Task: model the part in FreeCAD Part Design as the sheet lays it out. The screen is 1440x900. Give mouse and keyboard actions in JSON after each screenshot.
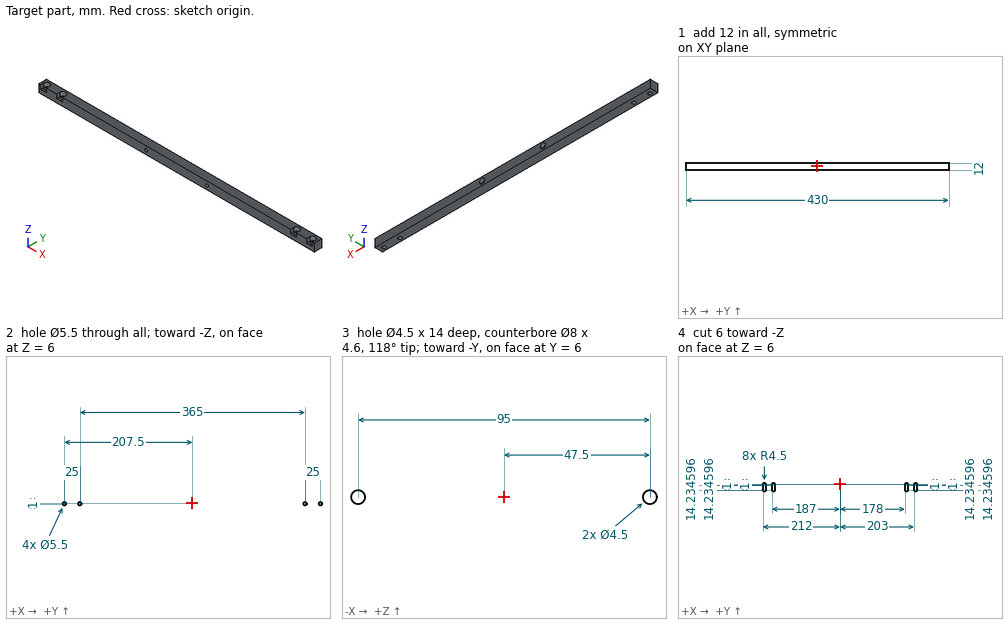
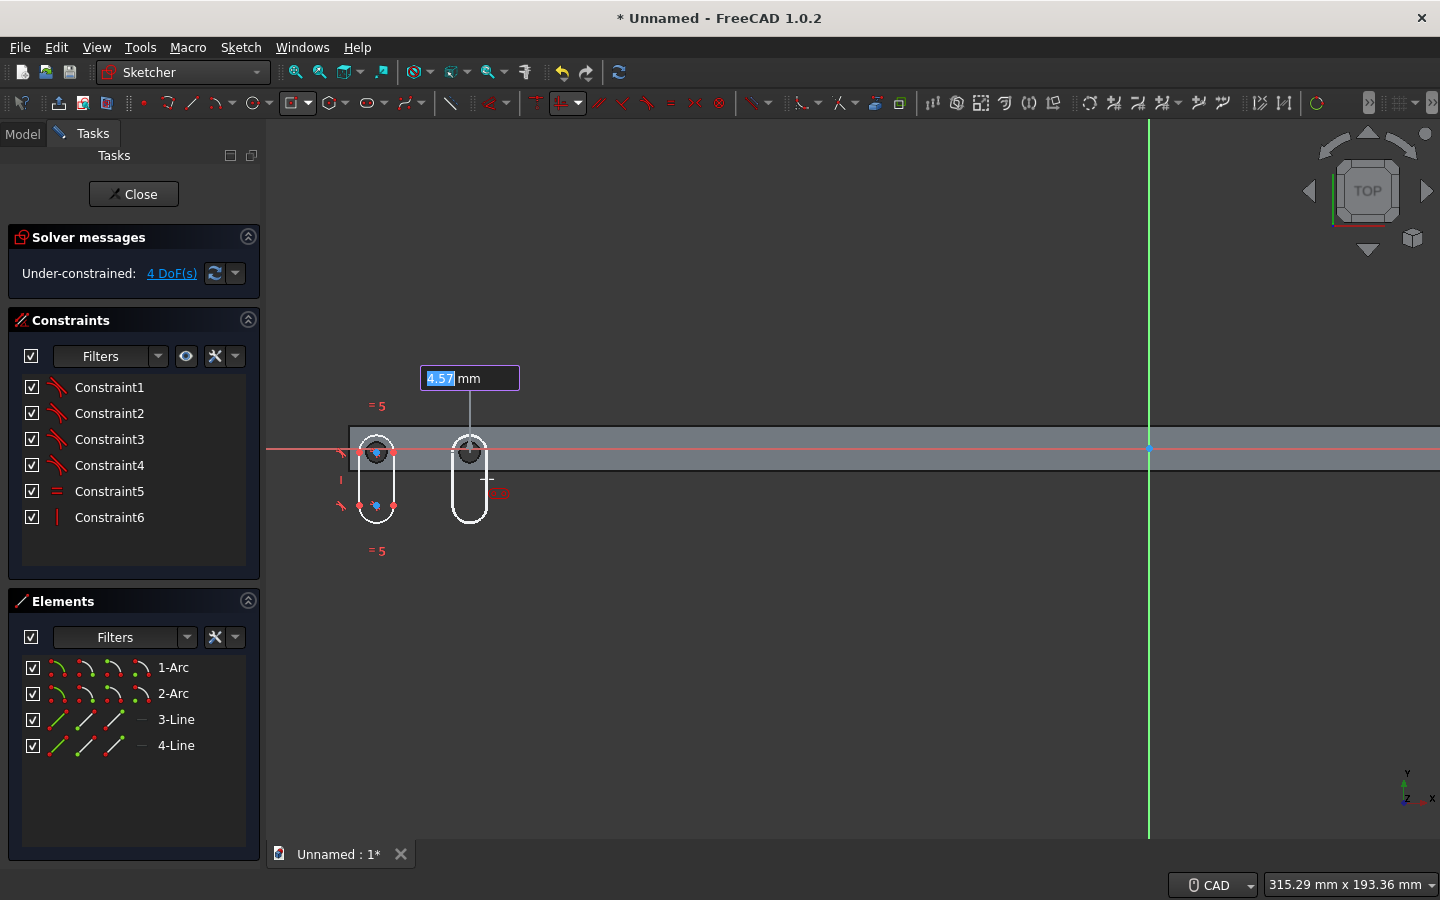
{"action": "left_click", "coordinate": [486, 479]}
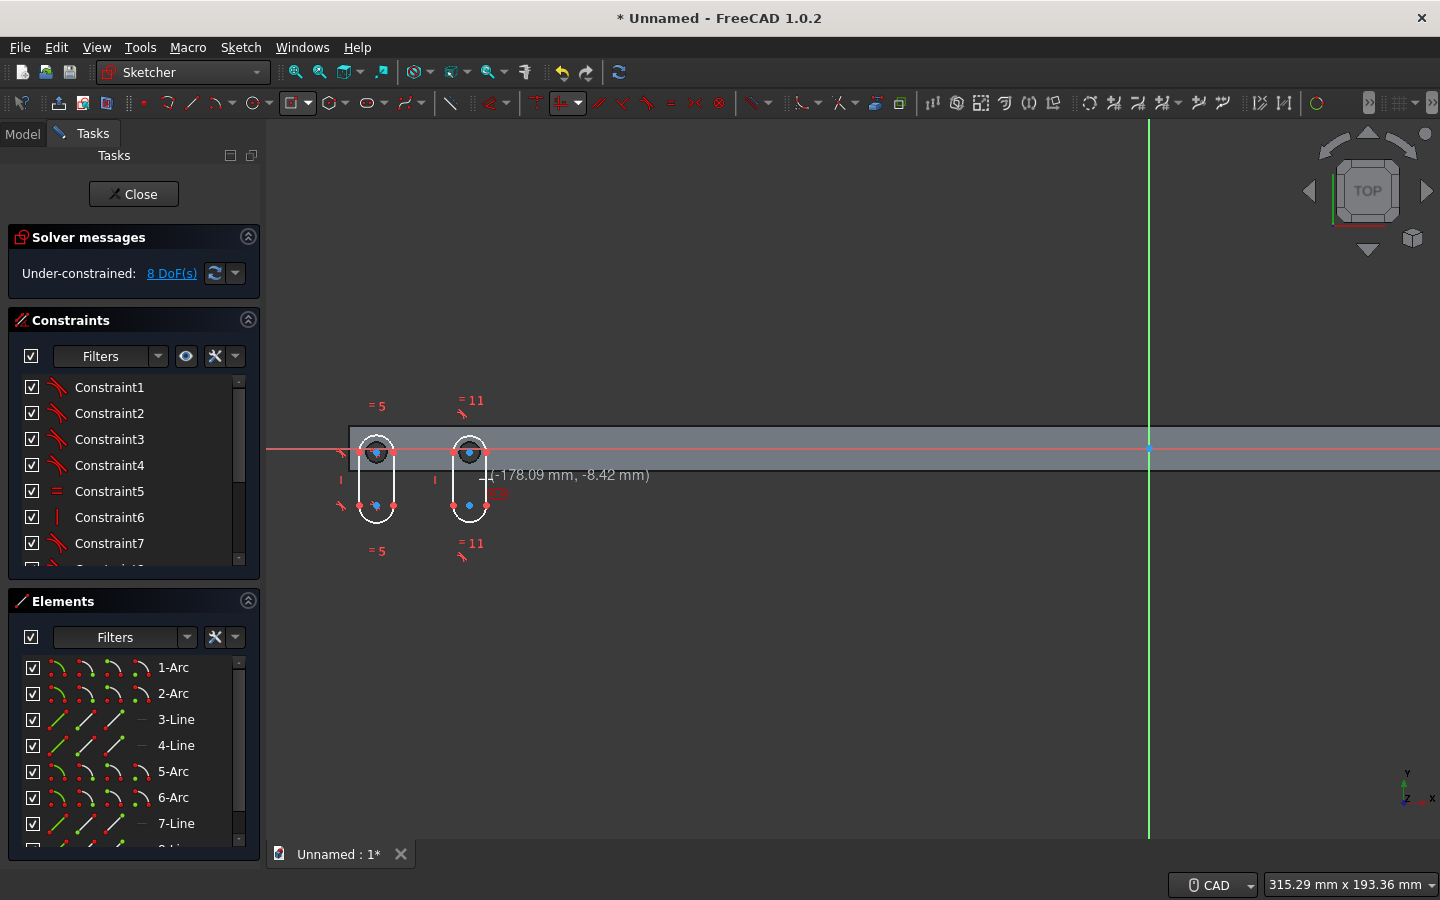
{"action": "scroll", "coordinate": [487, 479], "scroll_direction": "down", "scroll_amount": 4}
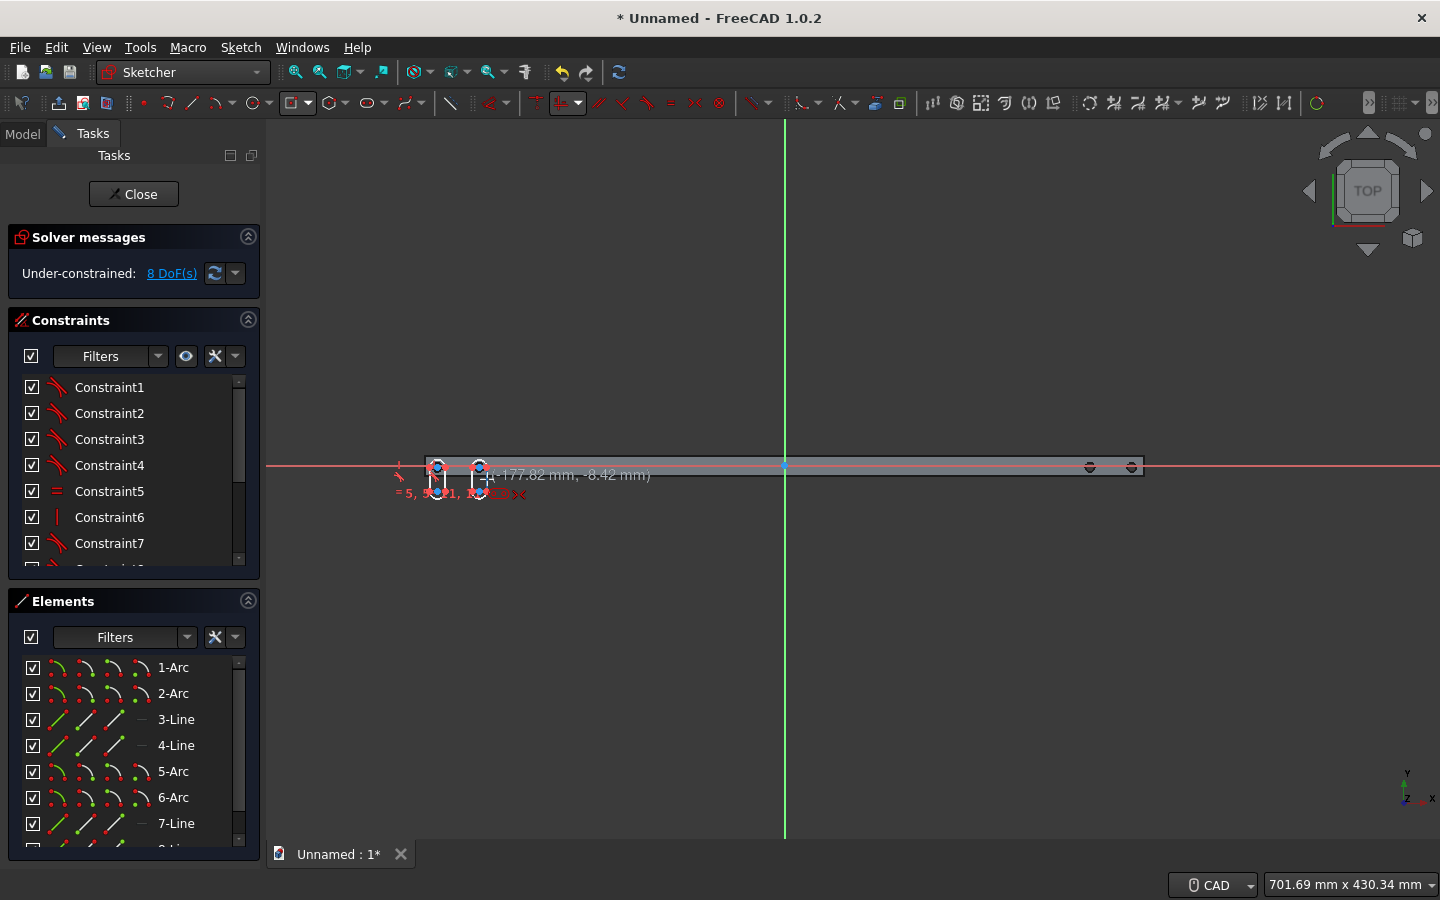
{"action": "scroll", "coordinate": [1090, 491], "scroll_direction": "up", "scroll_amount": 6}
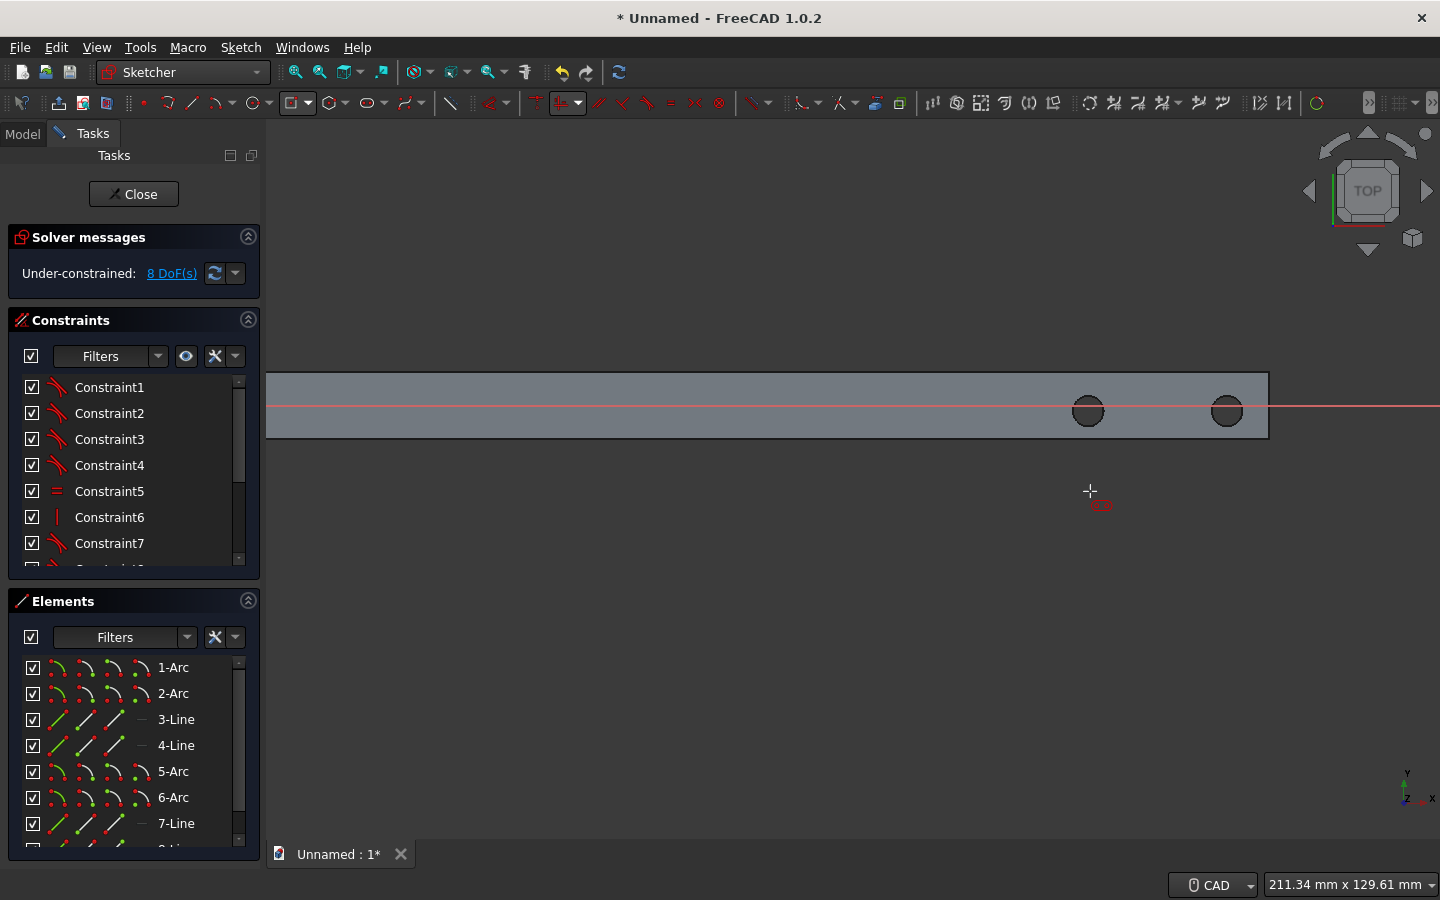
{"action": "left_click", "coordinate": [1088, 490]}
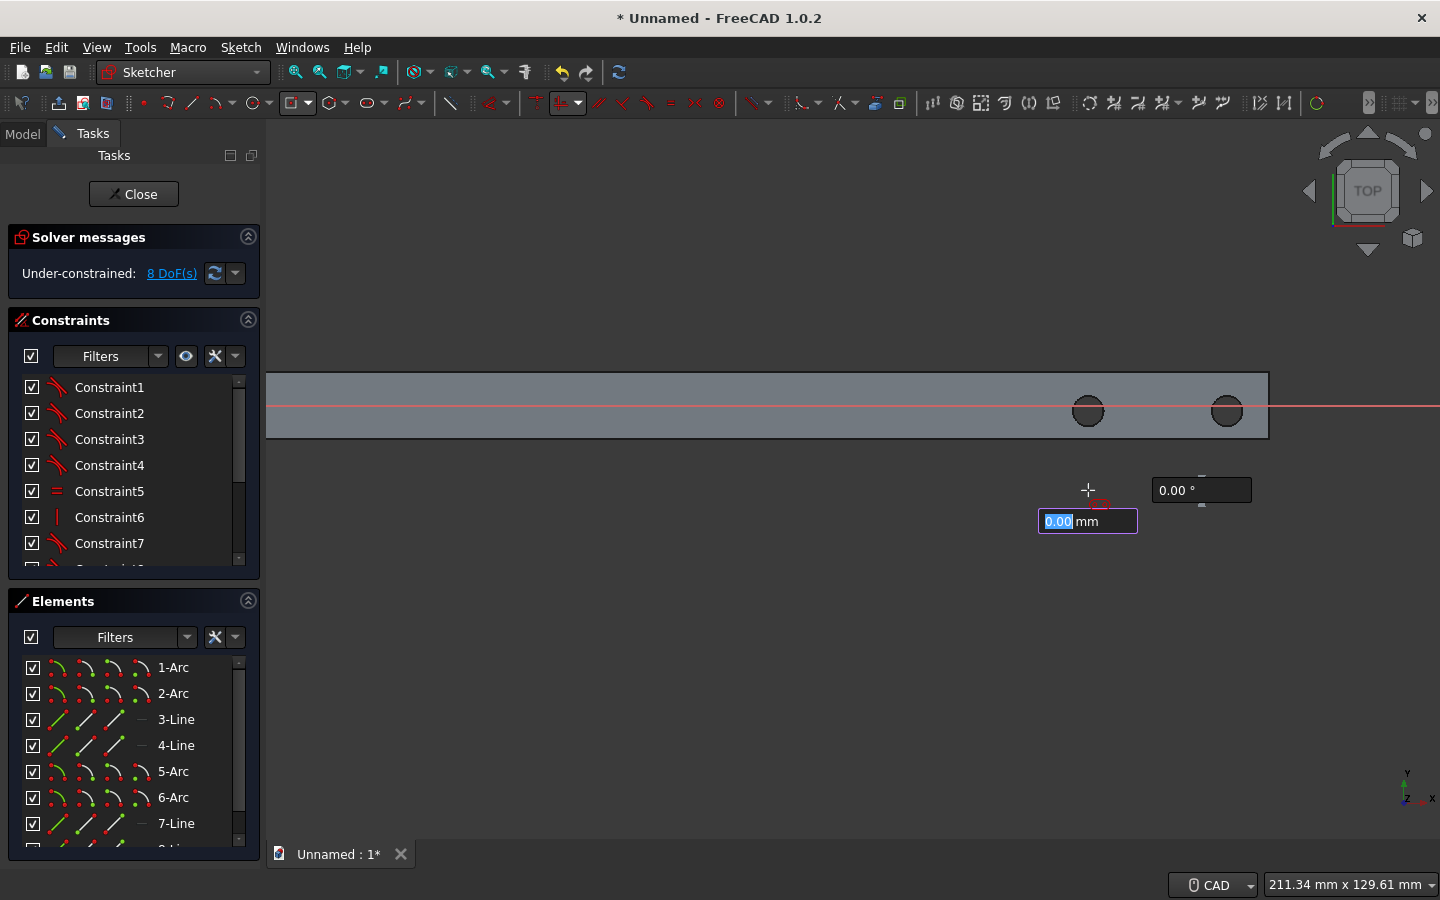
{"action": "scroll", "coordinate": [1088, 411], "scroll_direction": "up", "scroll_amount": 6}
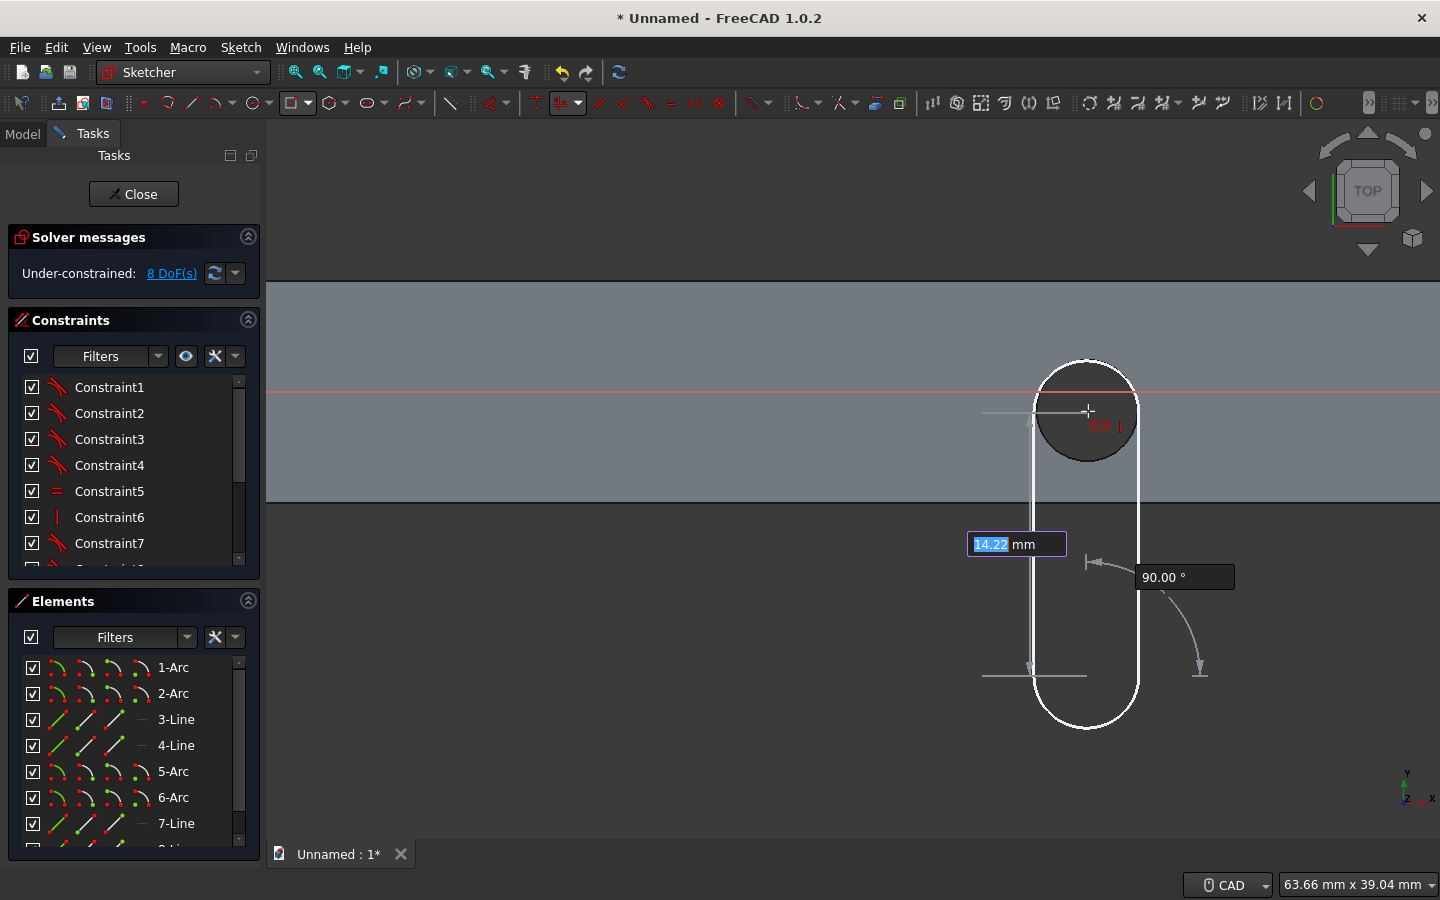
{"action": "left_click", "coordinate": [1086, 410]}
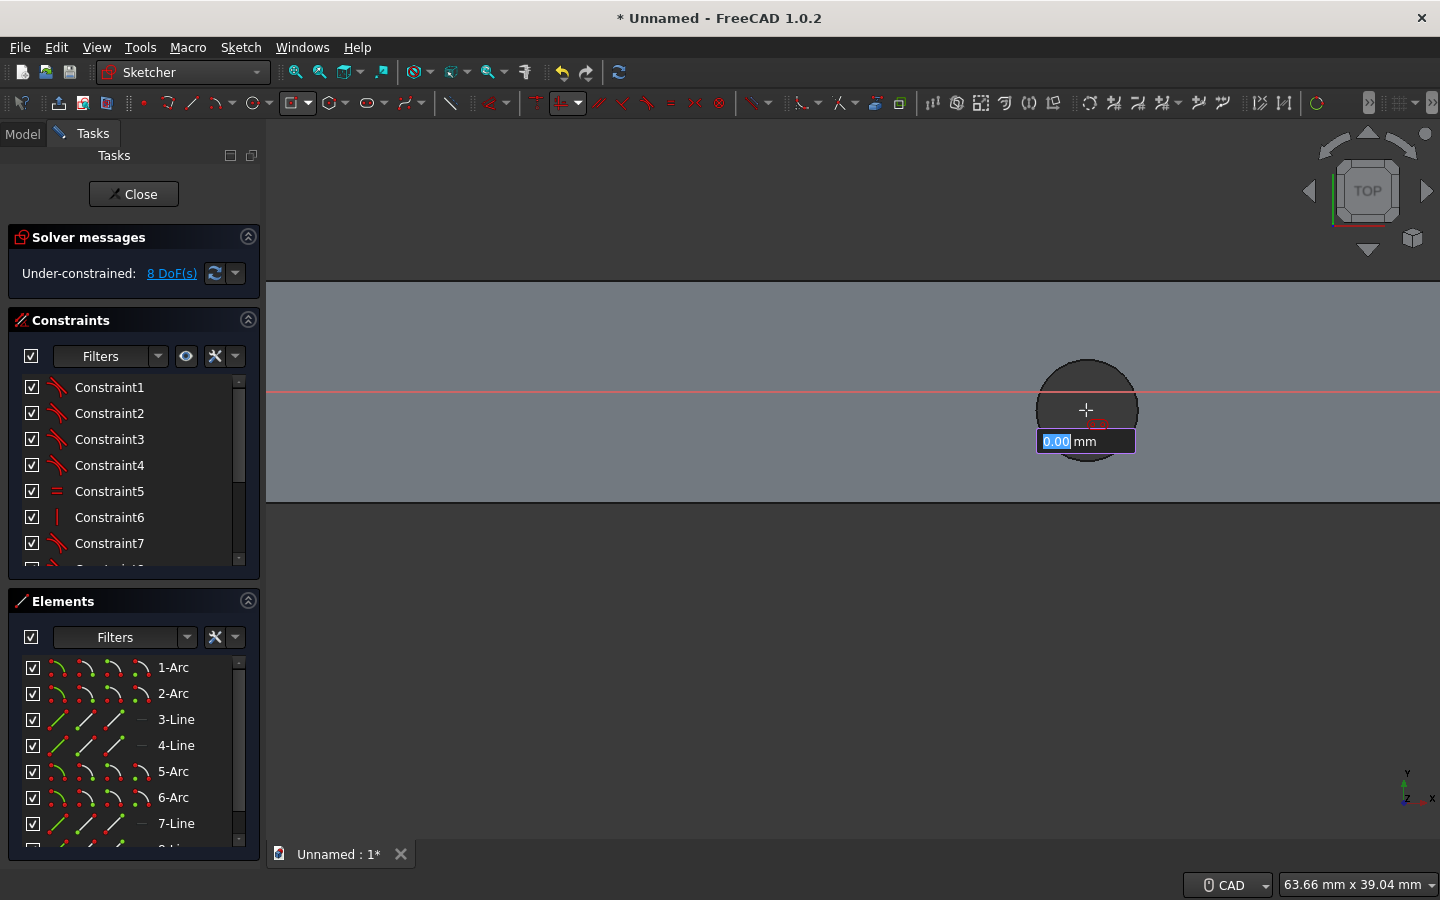
{"action": "scroll", "coordinate": [1090, 473], "scroll_direction": "down", "scroll_amount": 12}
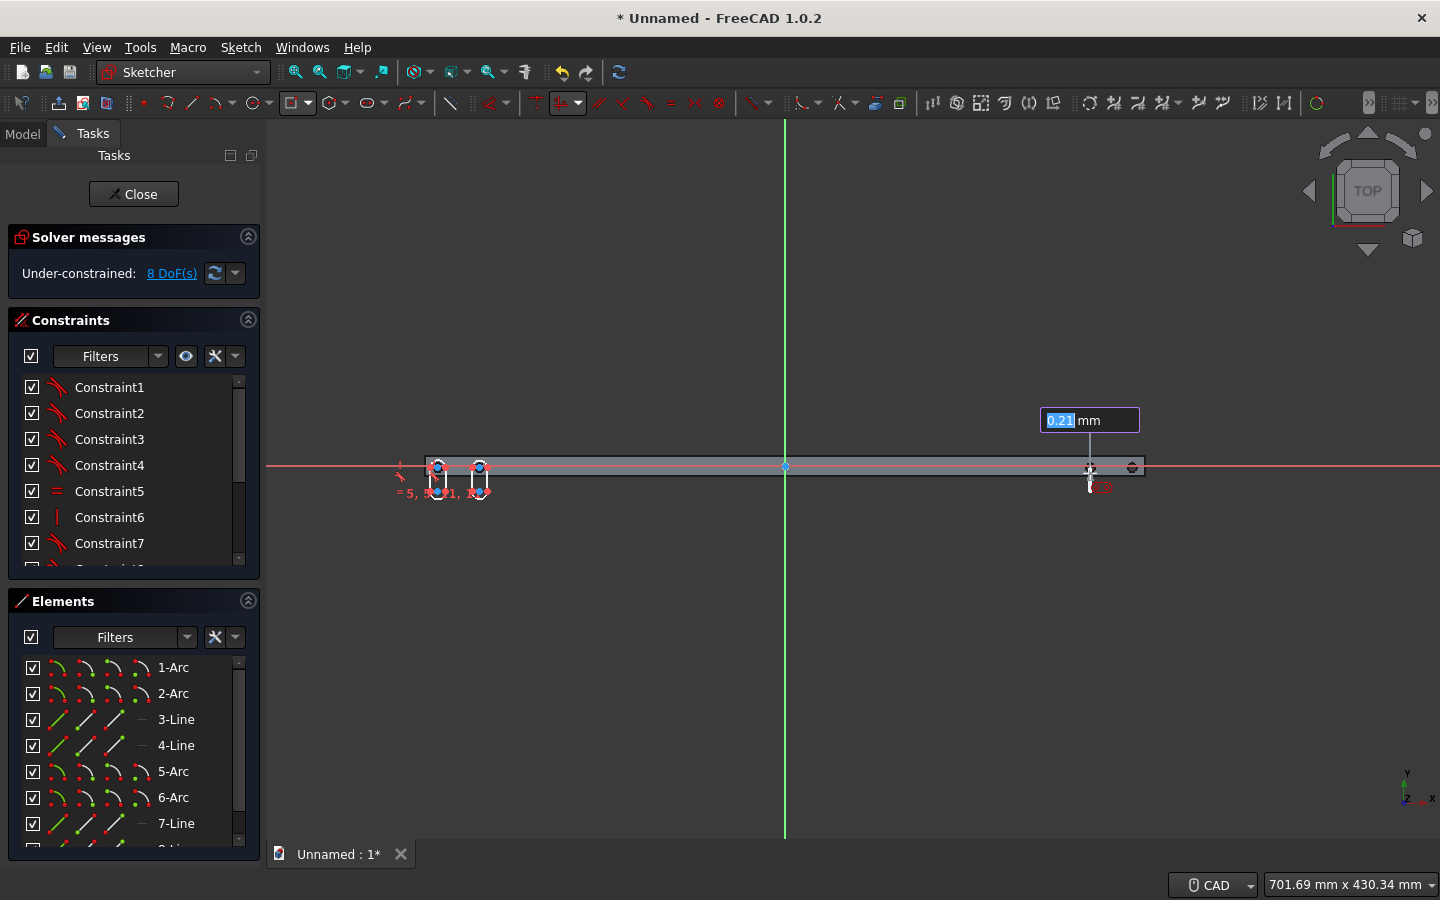
{"action": "scroll", "coordinate": [1098, 480], "scroll_direction": "up", "scroll_amount": 4}